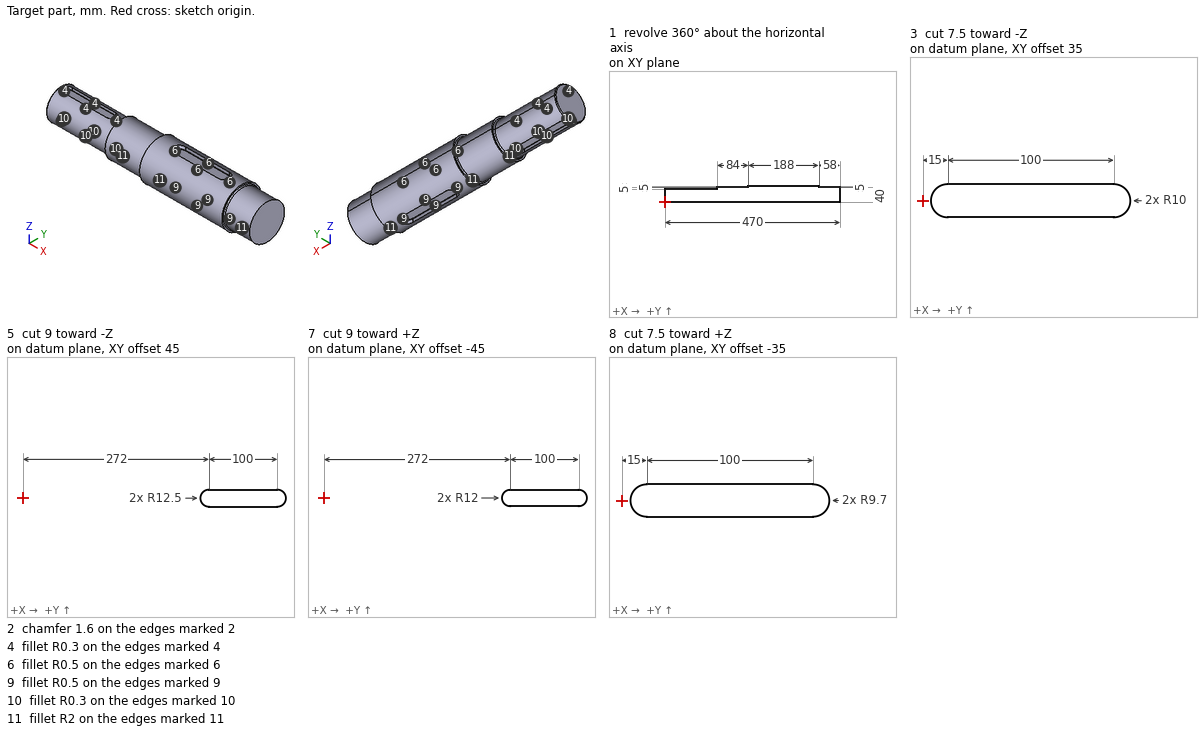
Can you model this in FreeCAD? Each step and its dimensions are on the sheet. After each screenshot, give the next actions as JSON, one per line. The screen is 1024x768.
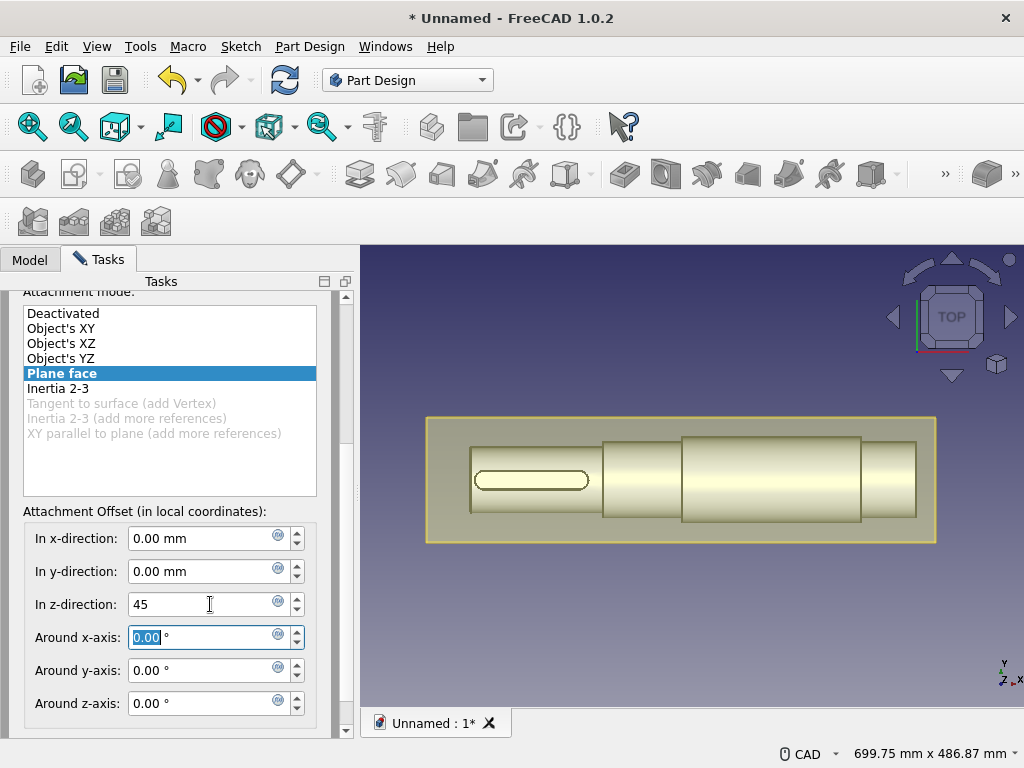
{"action": "scroll", "coordinate": [346, 514], "scroll_direction": "up", "scroll_amount": 5}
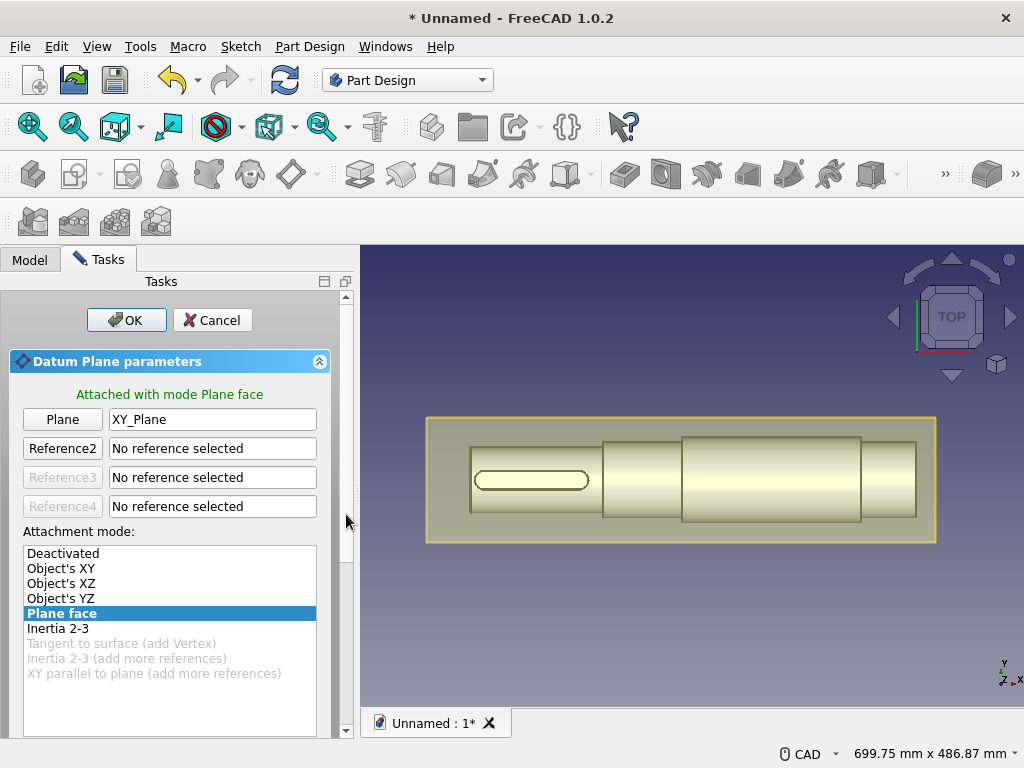
{"action": "left_click", "coordinate": [127, 320]}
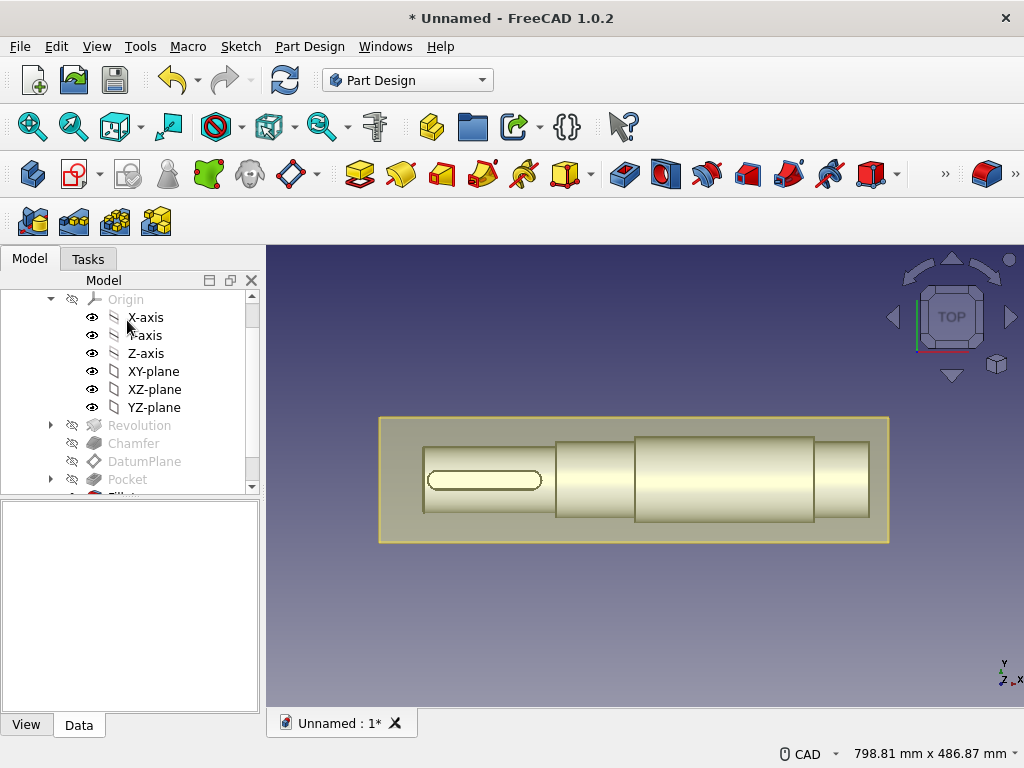
{"action": "scroll", "coordinate": [141, 385], "scroll_direction": "down", "scroll_amount": 3}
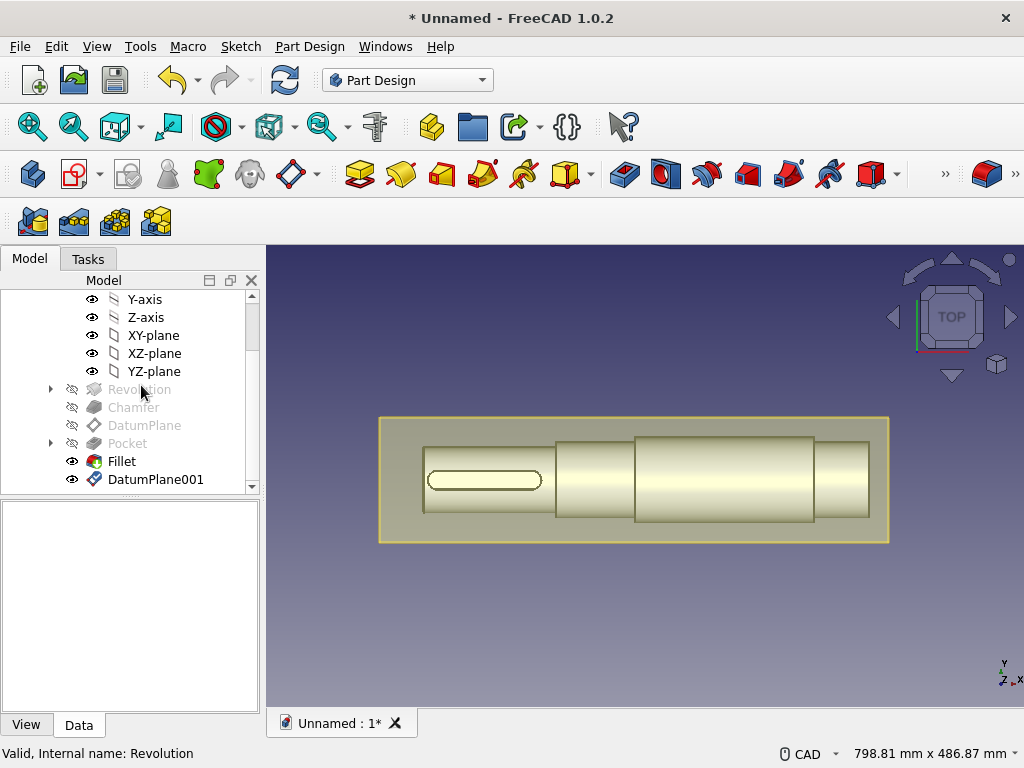
{"action": "left_click", "coordinate": [117, 479]}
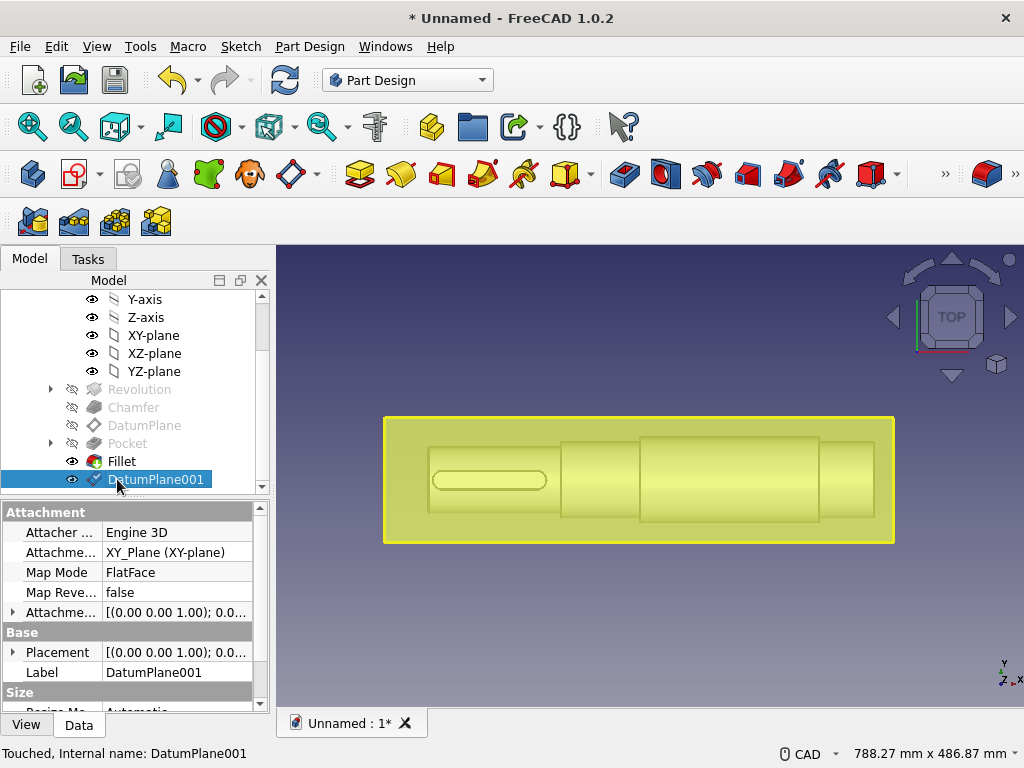
{"action": "left_click", "coordinate": [74, 174]}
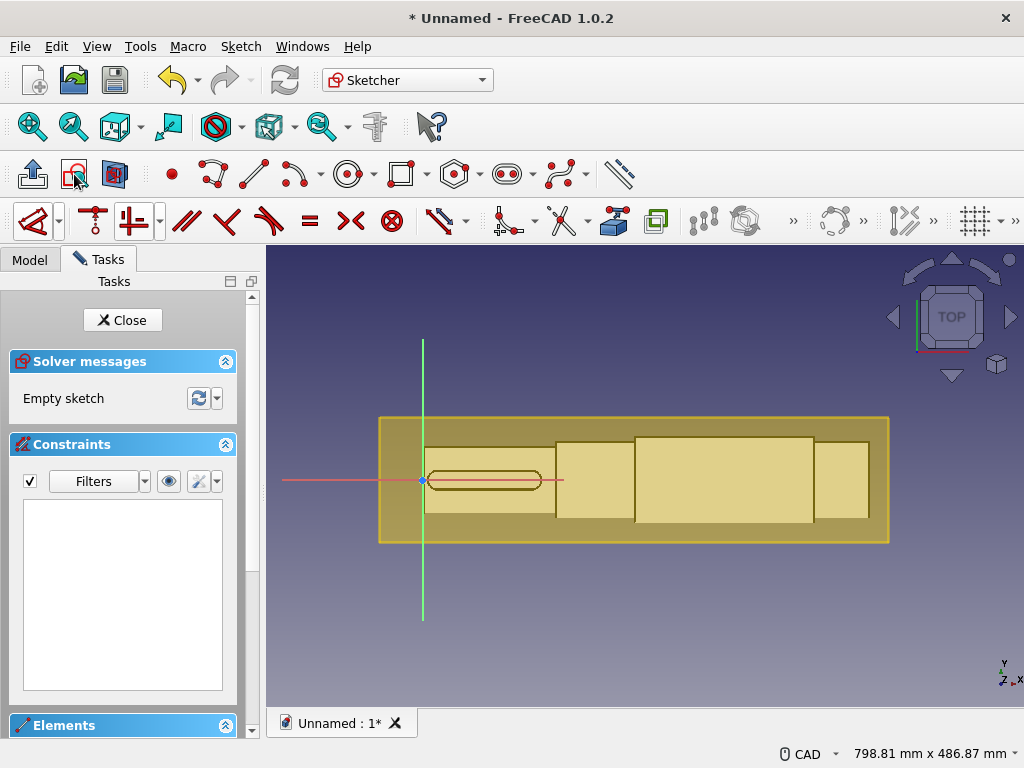
{"action": "scroll", "coordinate": [794, 482], "scroll_direction": "up", "scroll_amount": 6}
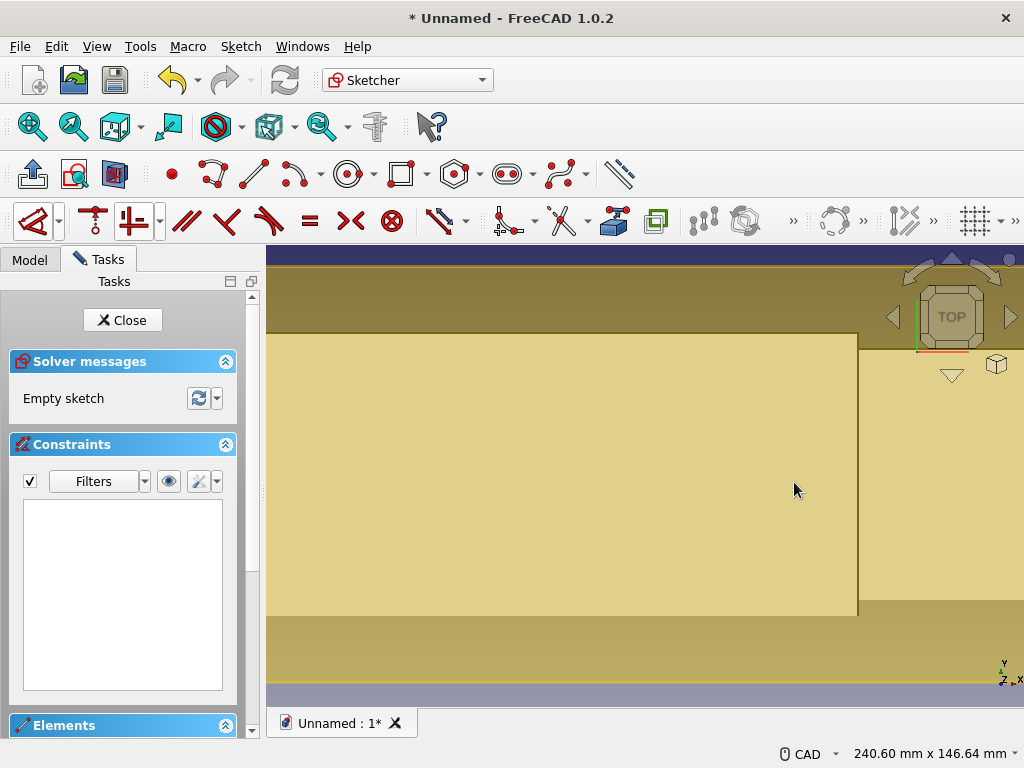
{"action": "left_click", "coordinate": [506, 174]}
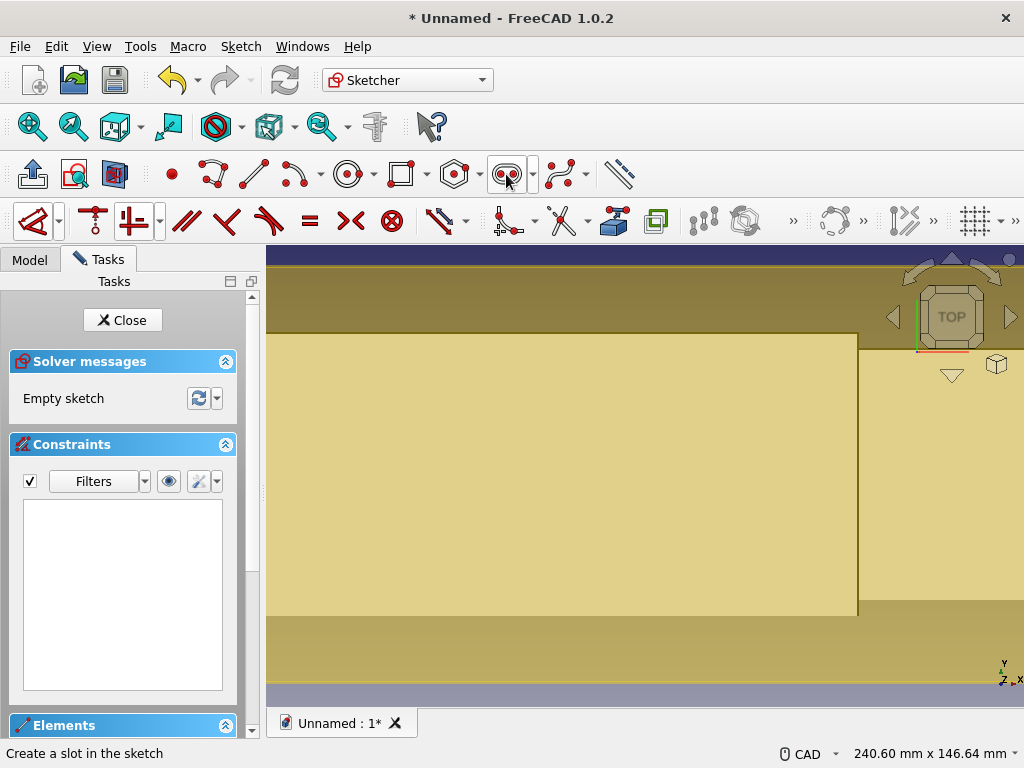
{"action": "left_click", "coordinate": [417, 475]}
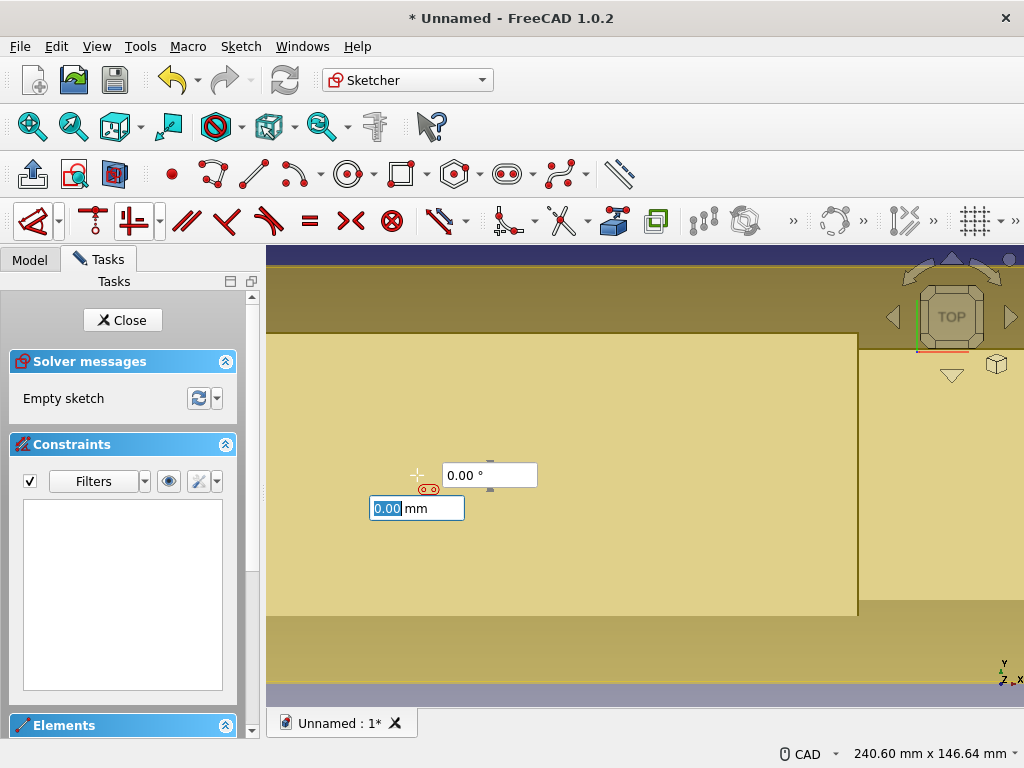
{"action": "left_click", "coordinate": [732, 466]}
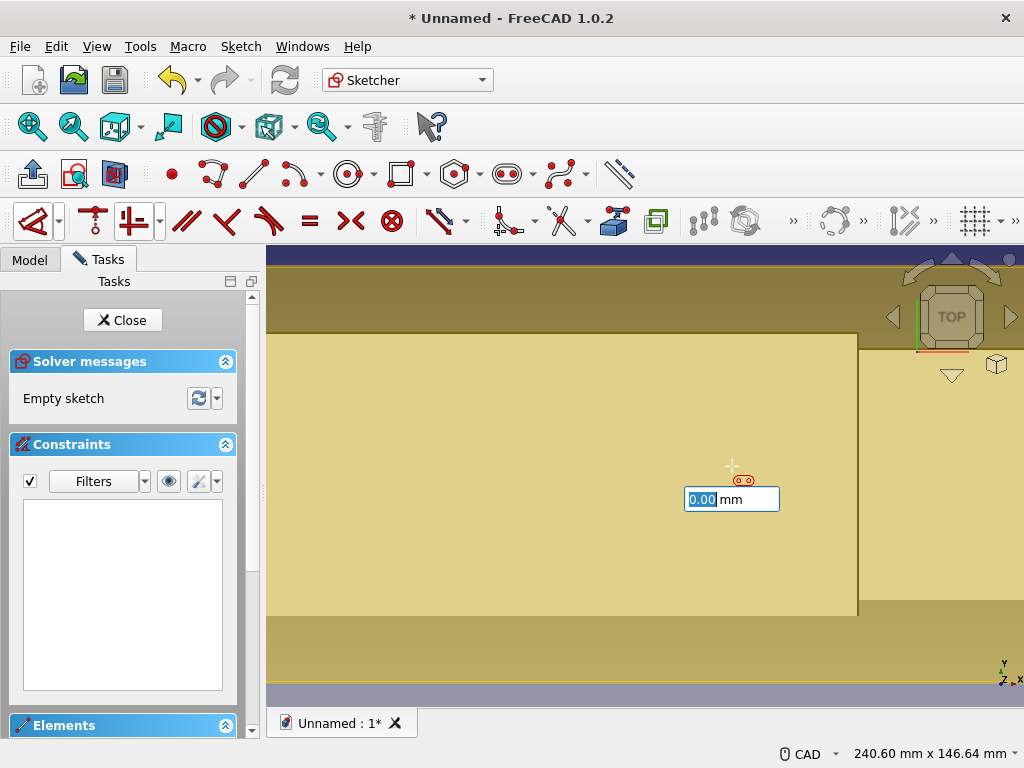
{"action": "left_click", "coordinate": [575, 435]}
{"action": "key", "text": "Escape"}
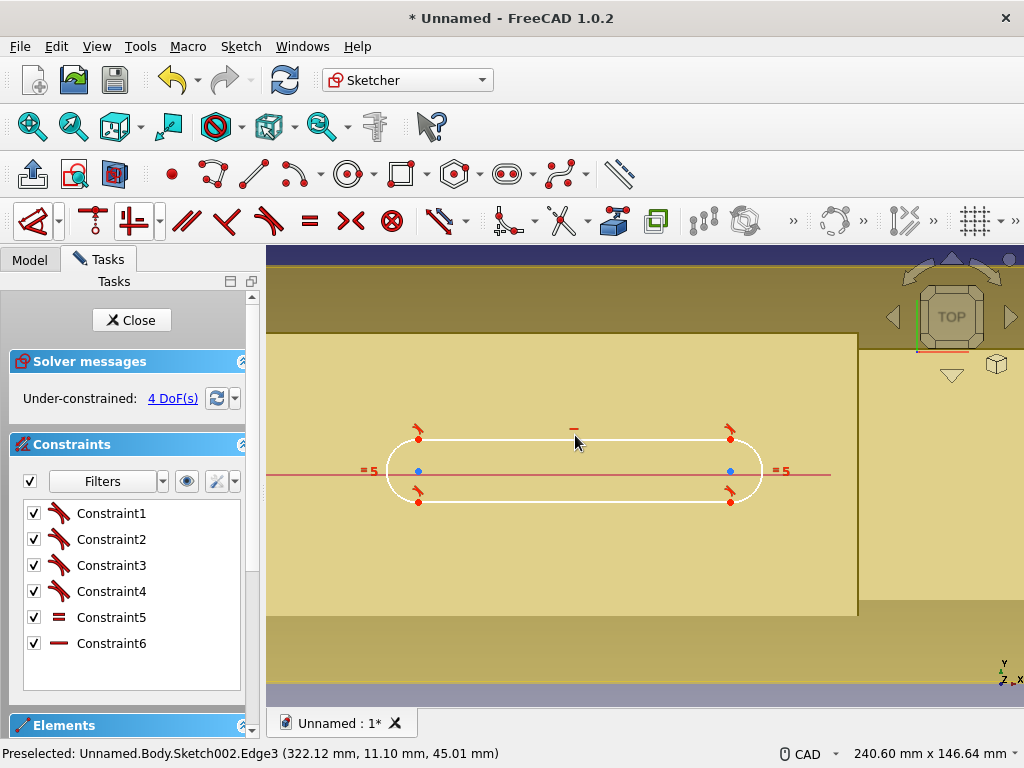
{"action": "left_click", "coordinate": [418, 471]}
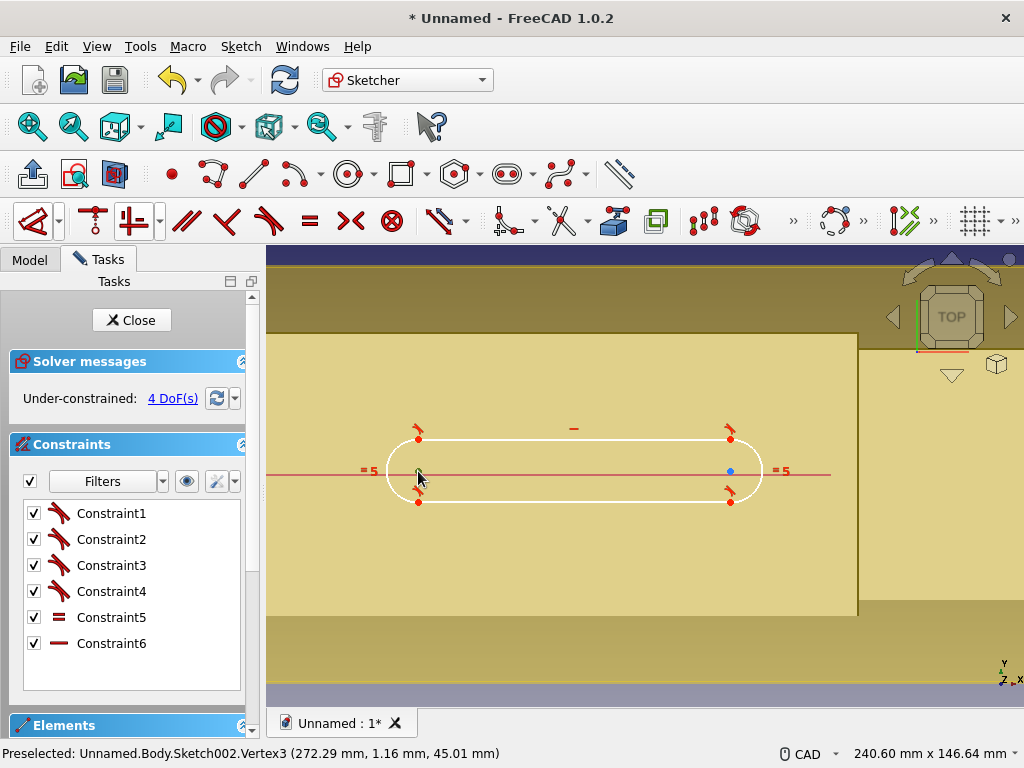
{"action": "left_click", "coordinate": [334, 475]}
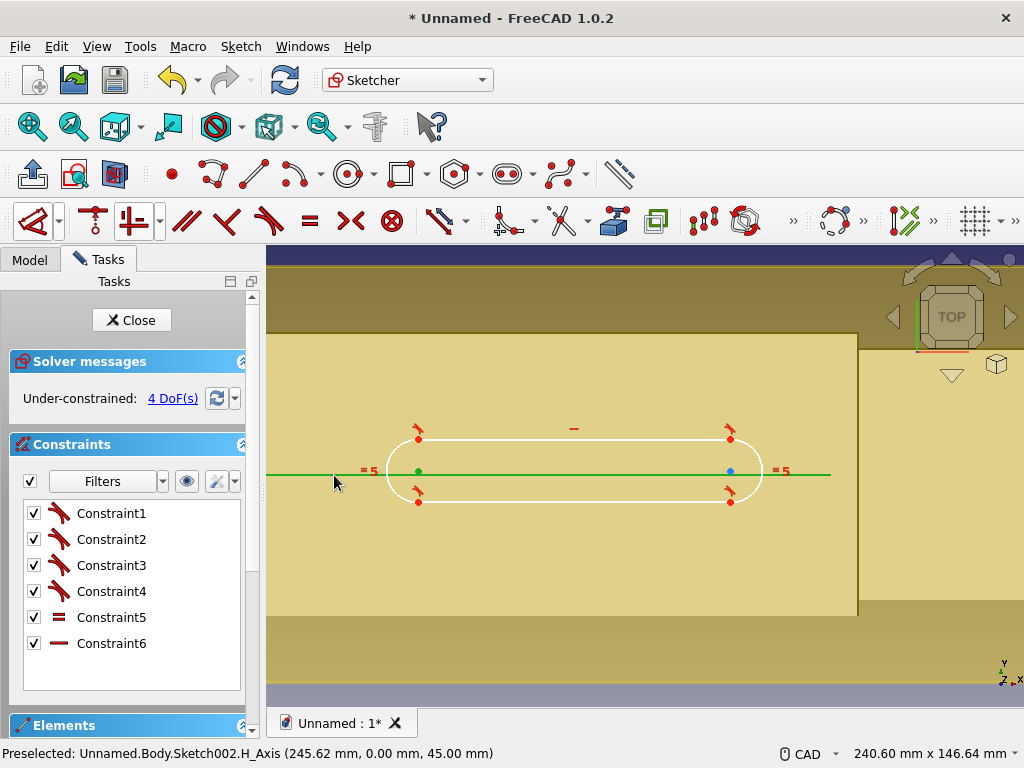
{"action": "left_click", "coordinate": [93, 222]}